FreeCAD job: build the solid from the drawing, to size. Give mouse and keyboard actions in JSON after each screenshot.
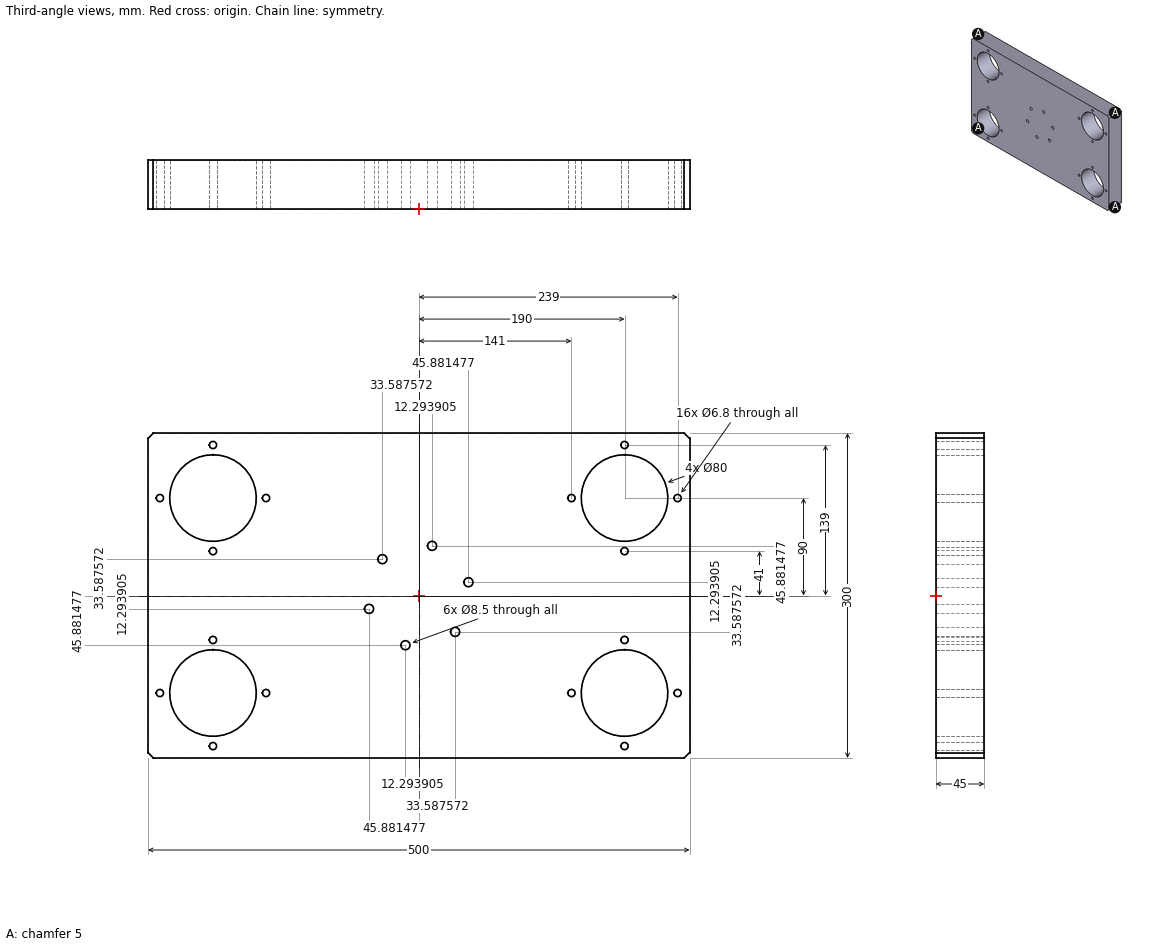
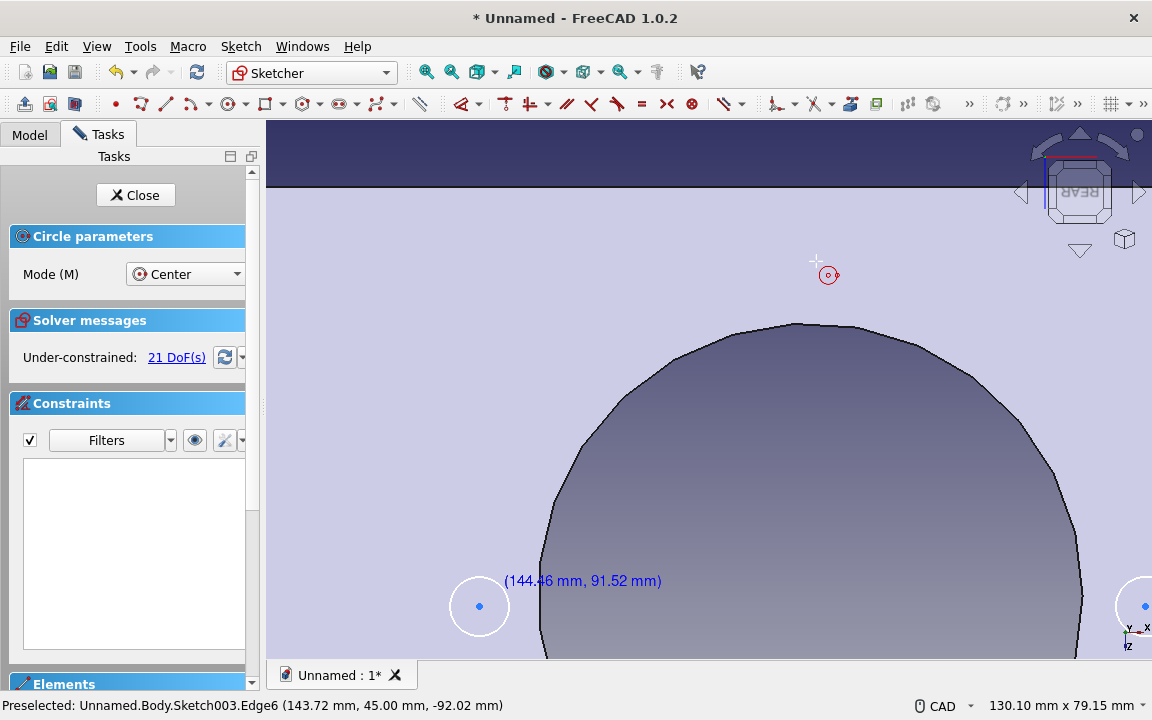
{"action": "scroll", "coordinate": [816, 261], "scroll_direction": "down", "scroll_amount": 10}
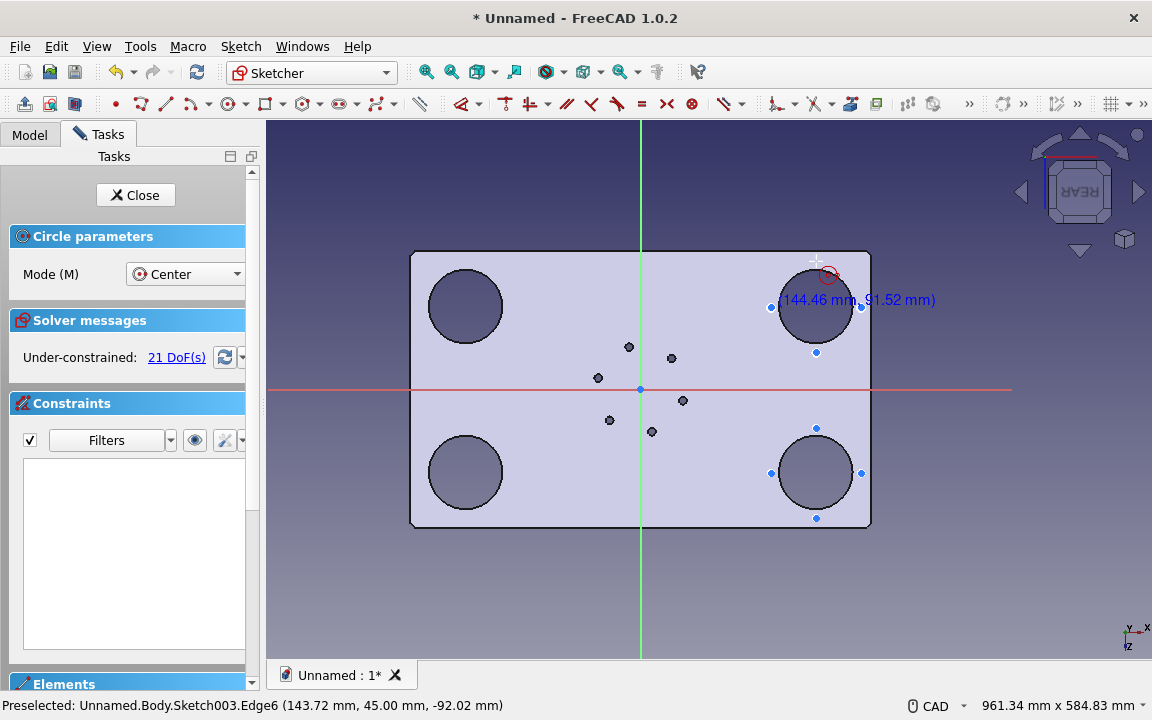
{"action": "left_click", "coordinate": [816, 261]}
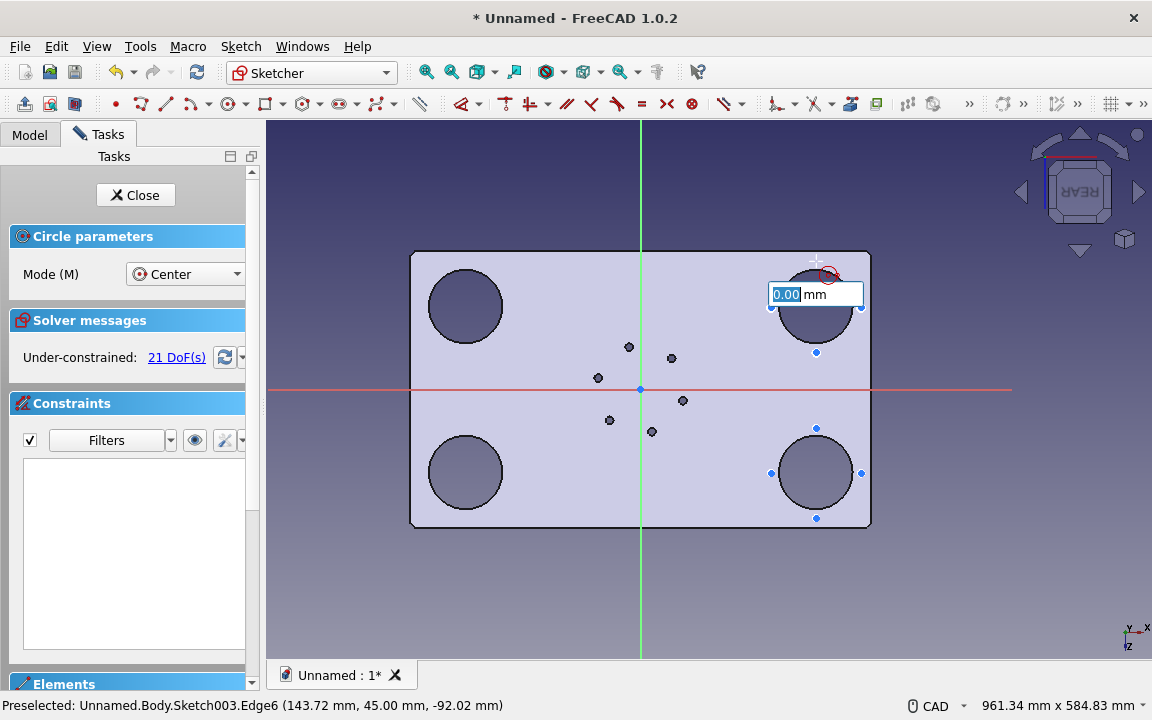
{"action": "scroll", "coordinate": [818, 259], "scroll_direction": "up", "scroll_amount": 9}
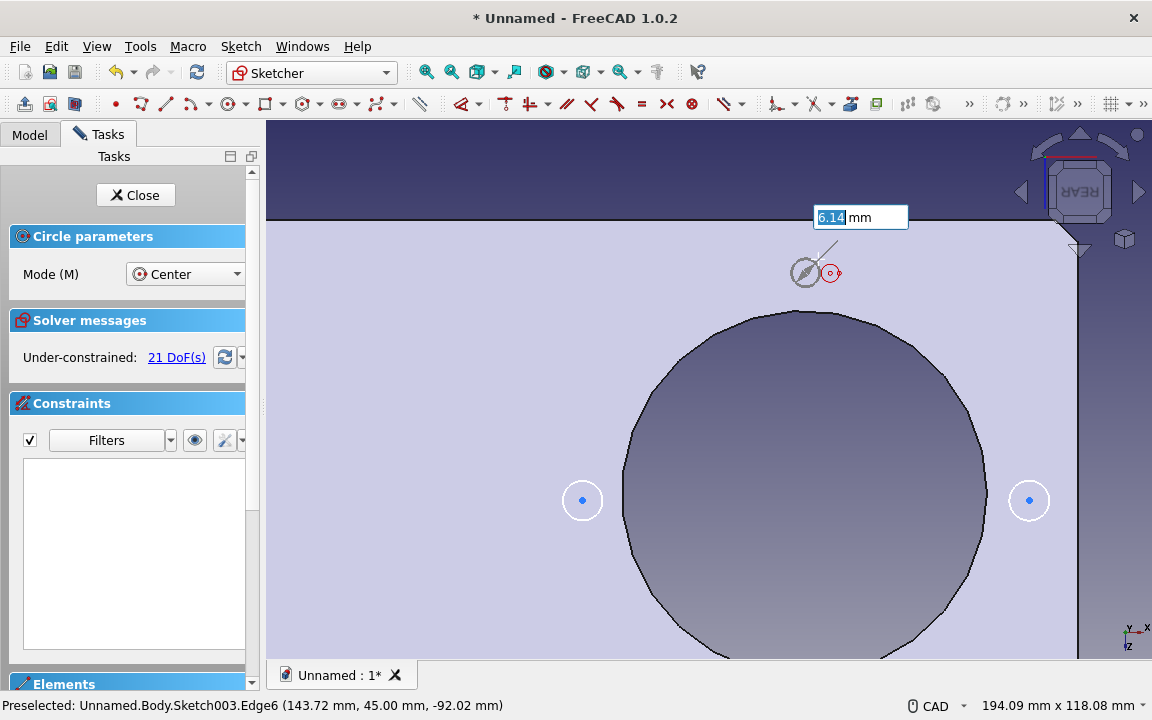
{"action": "left_click", "coordinate": [815, 259]}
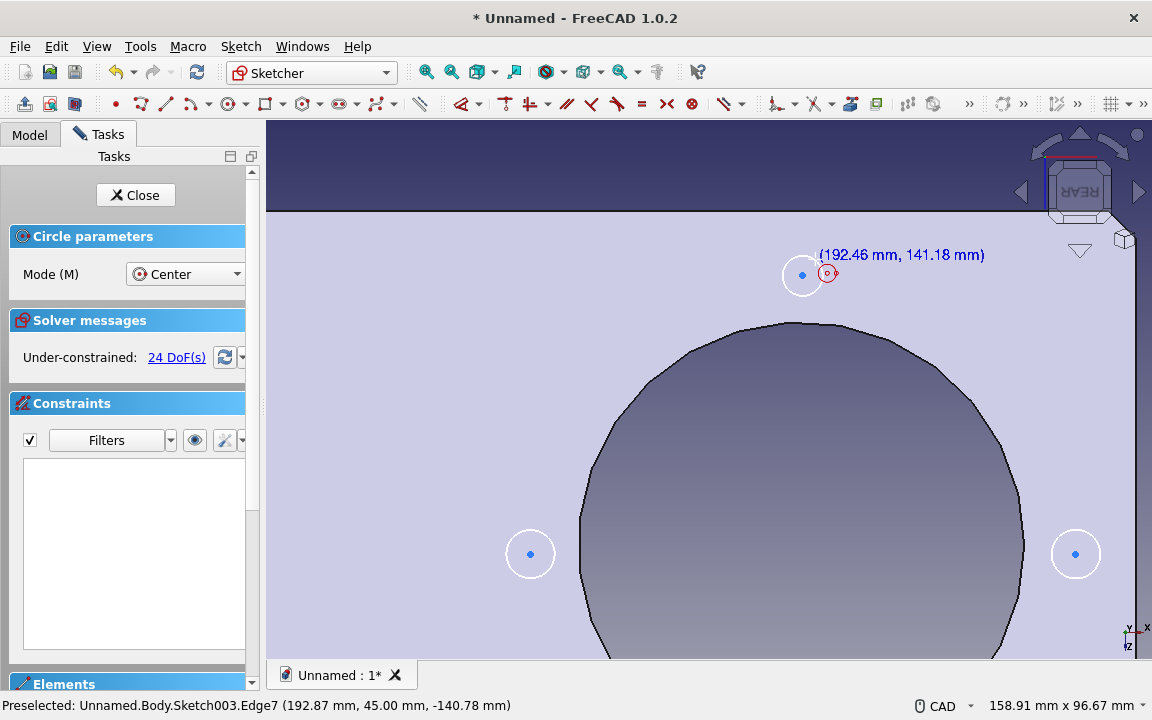
{"action": "scroll", "coordinate": [818, 259], "scroll_direction": "down", "scroll_amount": 9}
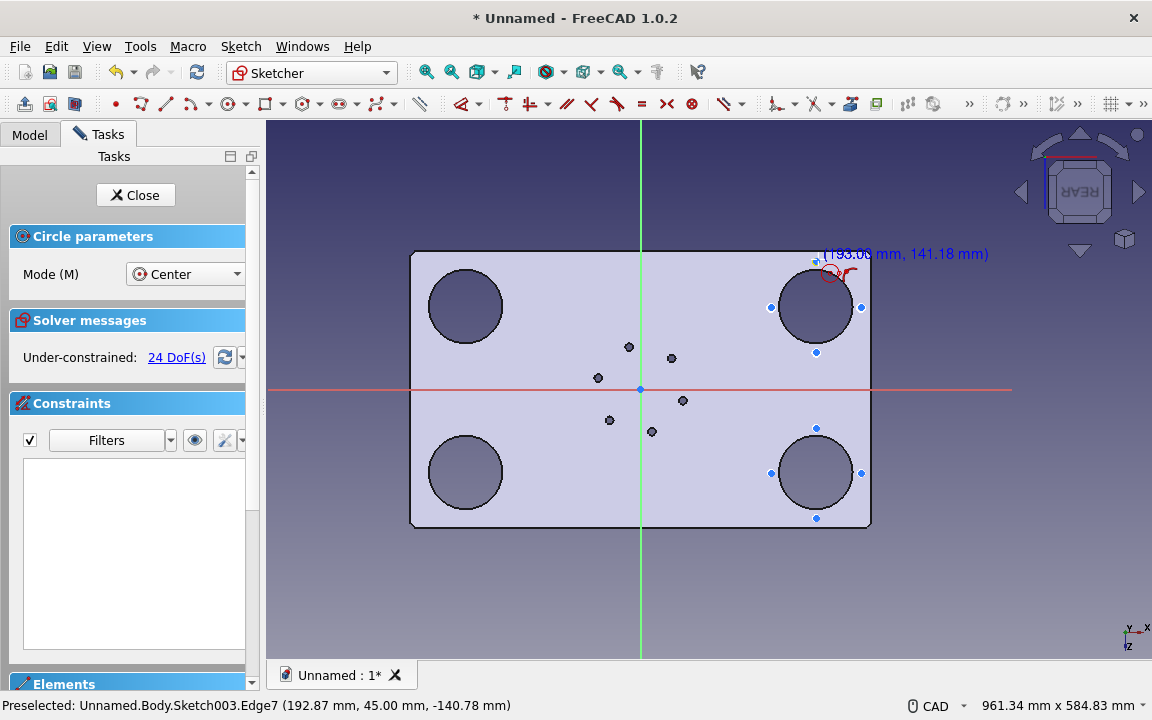
{"action": "scroll", "coordinate": [511, 472], "scroll_direction": "up", "scroll_amount": 10}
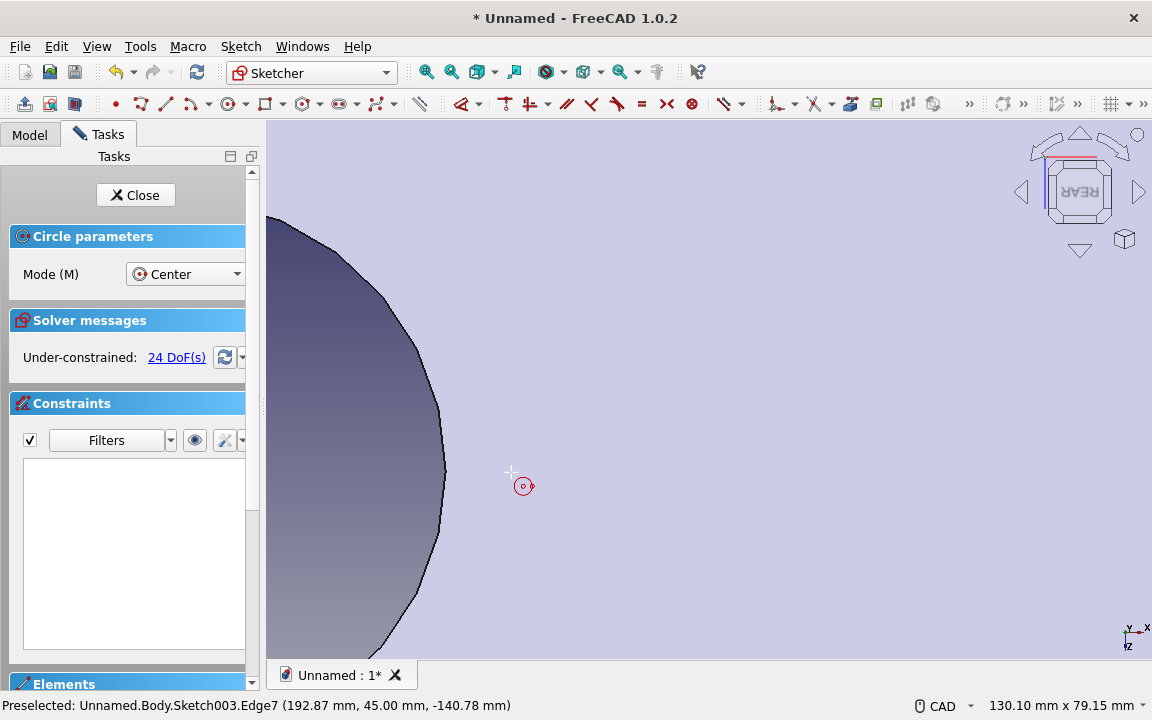
{"action": "scroll", "coordinate": [511, 473], "scroll_direction": "down", "scroll_amount": 10}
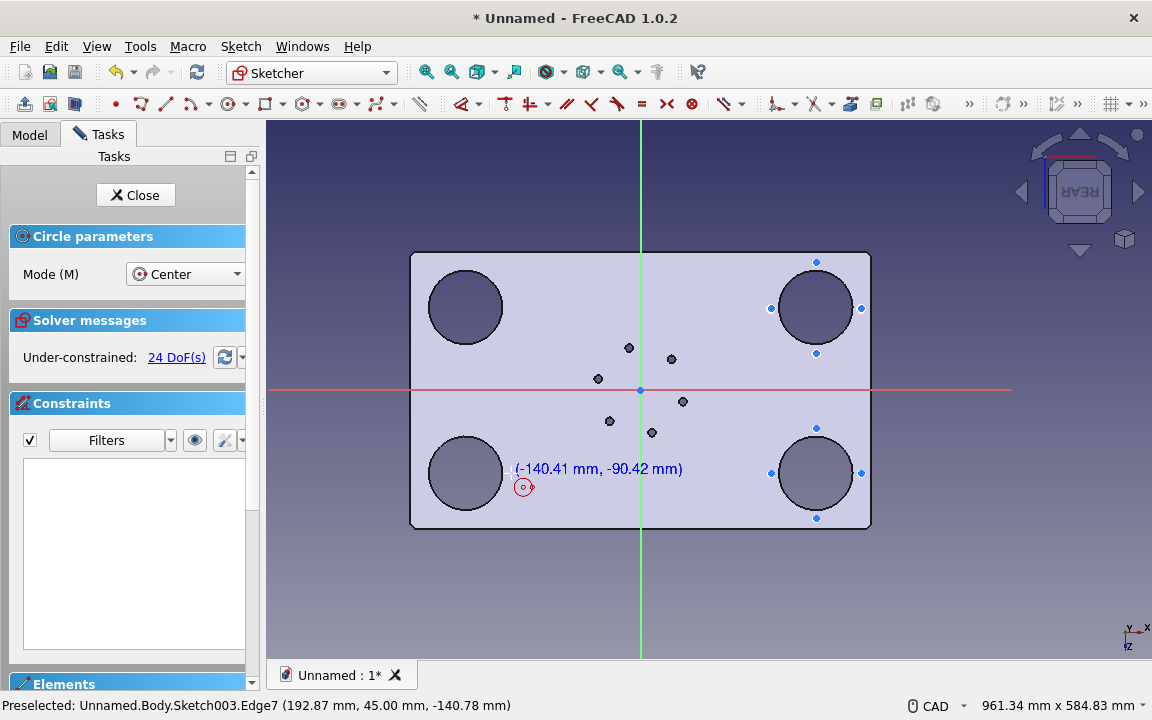
{"action": "left_click", "coordinate": [511, 473]}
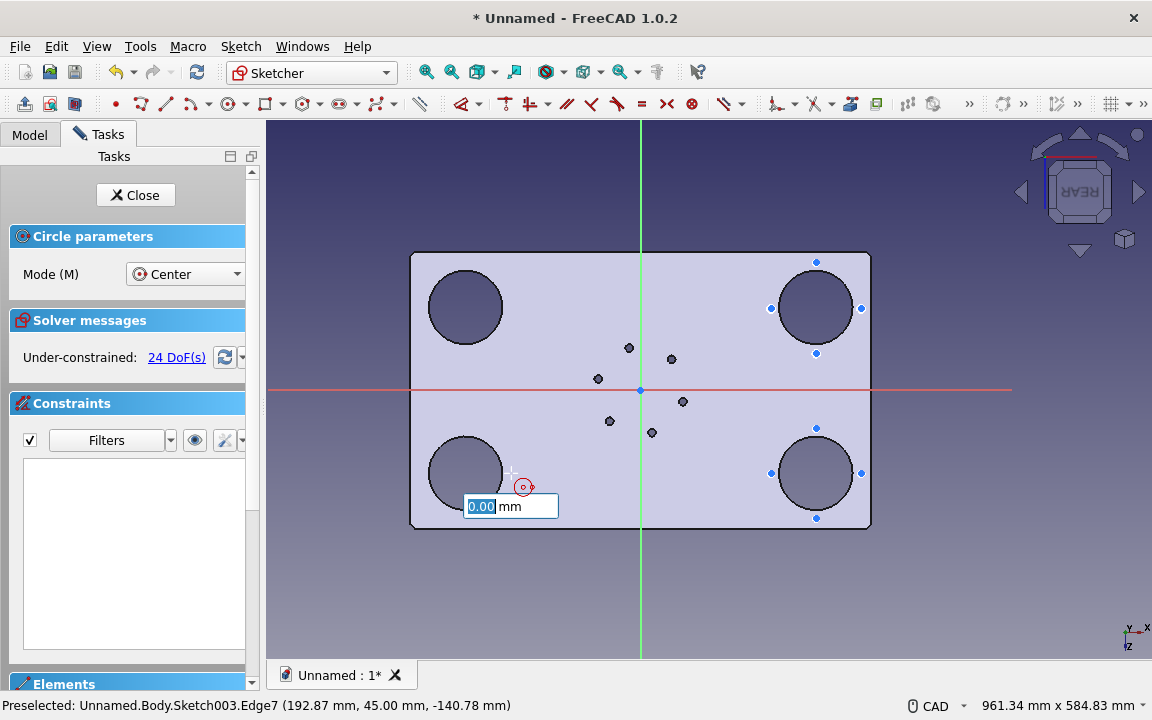
{"action": "scroll", "coordinate": [513, 471], "scroll_direction": "up", "scroll_amount": 9}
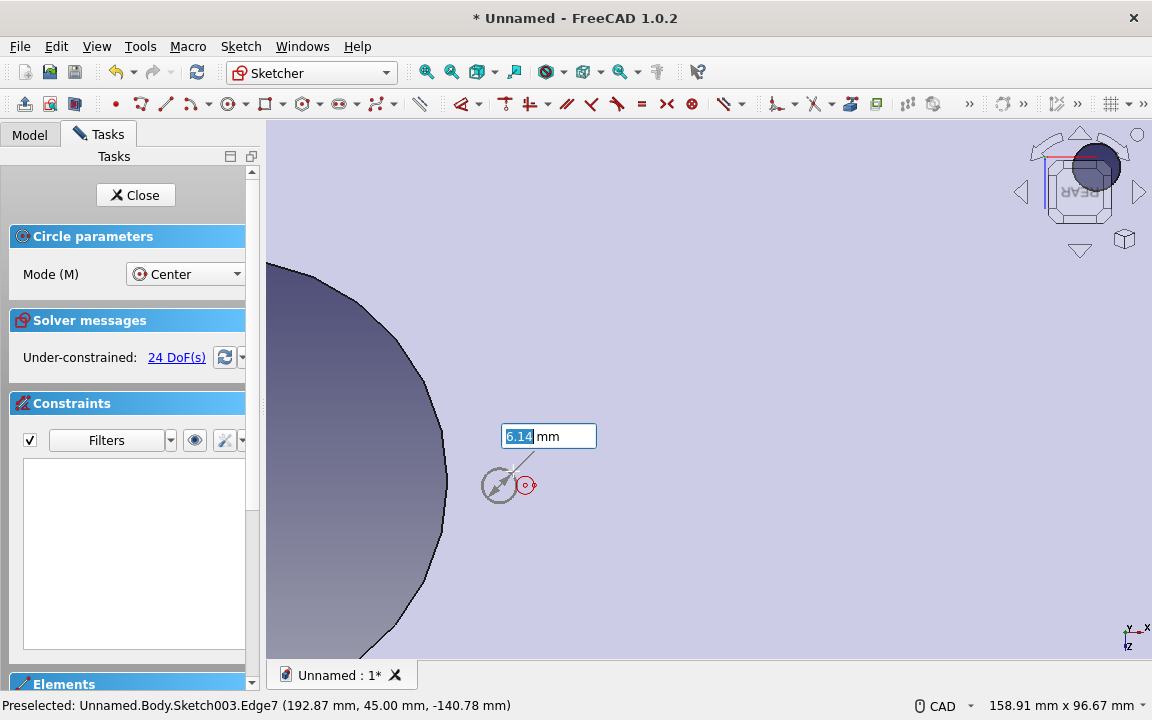
{"action": "left_click", "coordinate": [511, 468]}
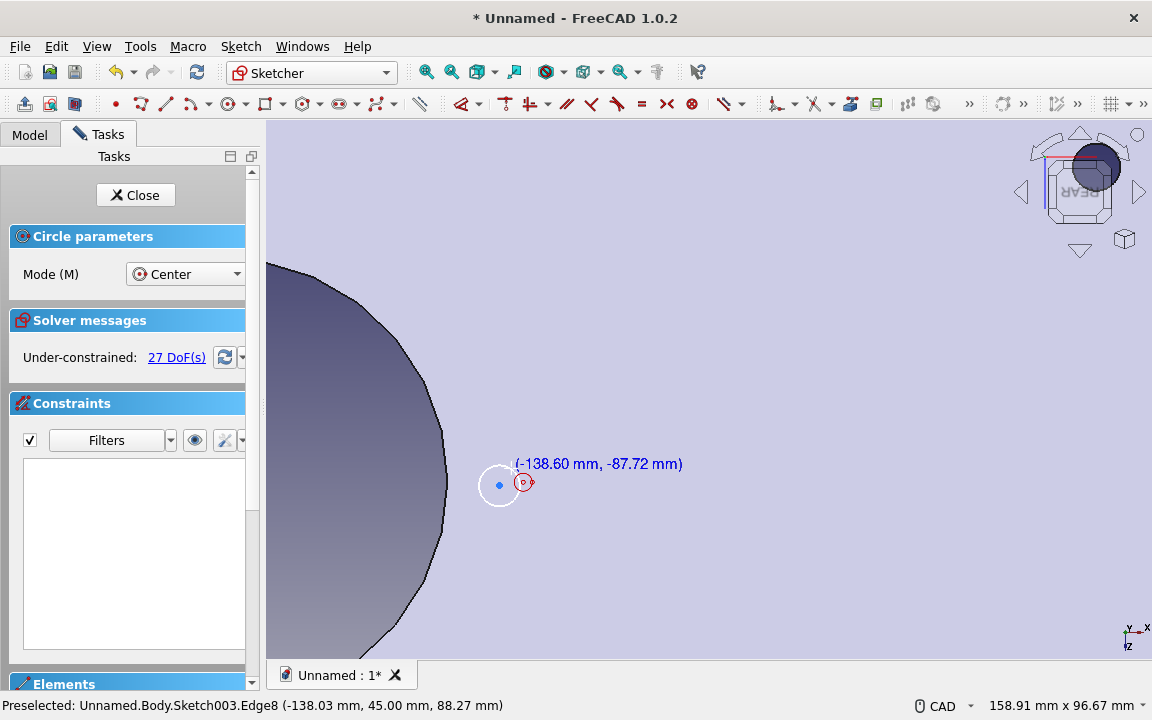
{"action": "scroll", "coordinate": [513, 471], "scroll_direction": "down", "scroll_amount": 9}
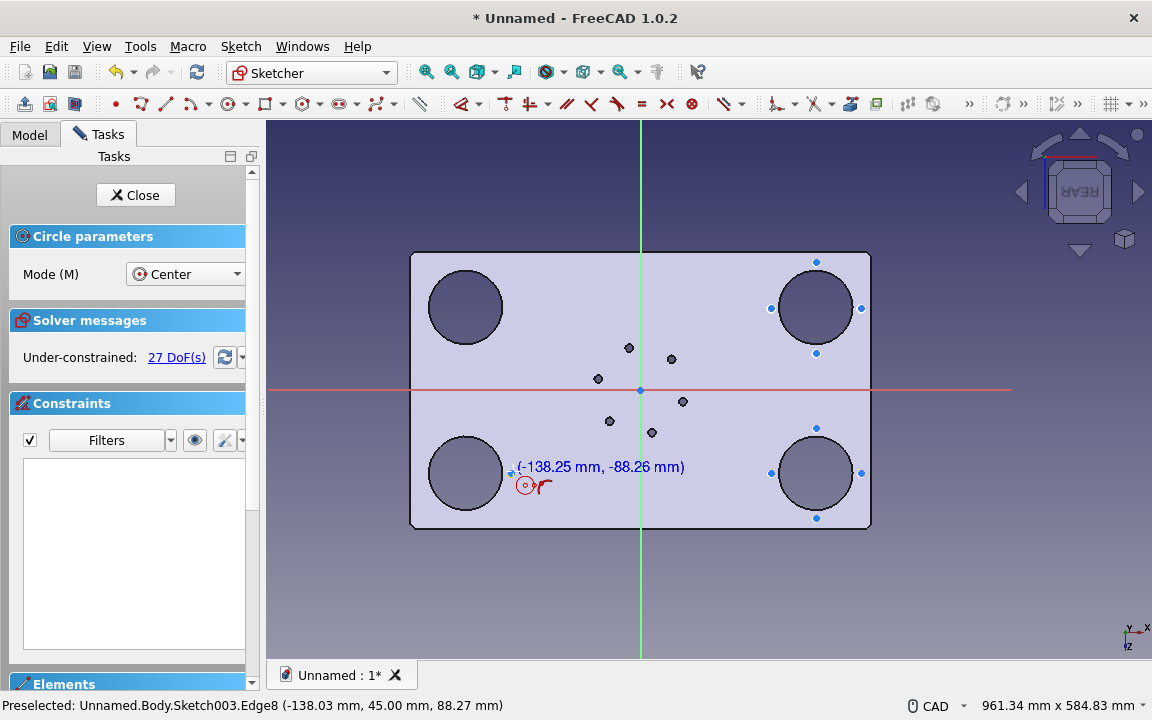
{"action": "scroll", "coordinate": [466, 518], "scroll_direction": "up", "scroll_amount": 10}